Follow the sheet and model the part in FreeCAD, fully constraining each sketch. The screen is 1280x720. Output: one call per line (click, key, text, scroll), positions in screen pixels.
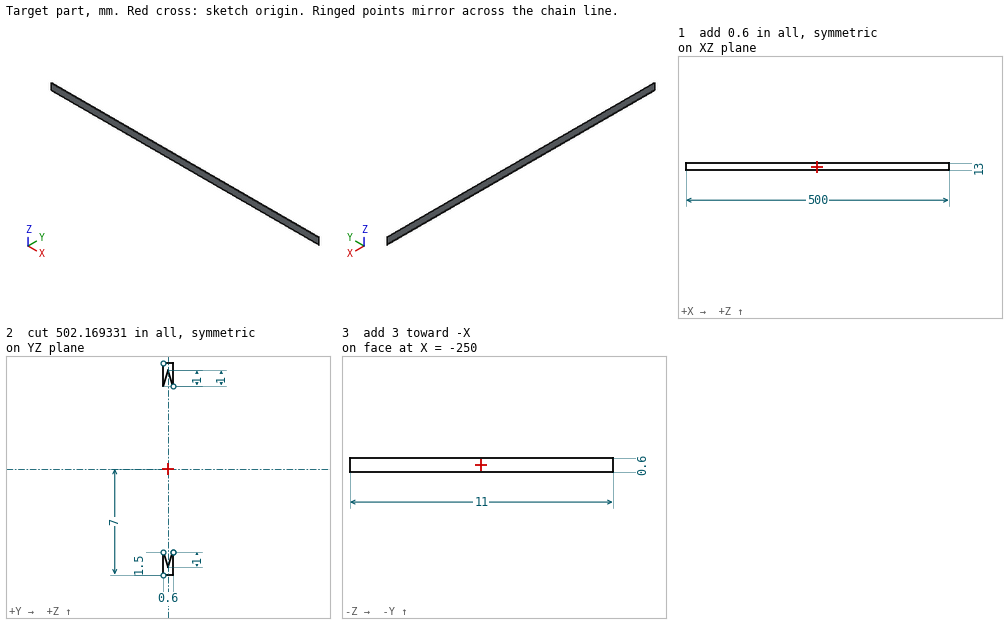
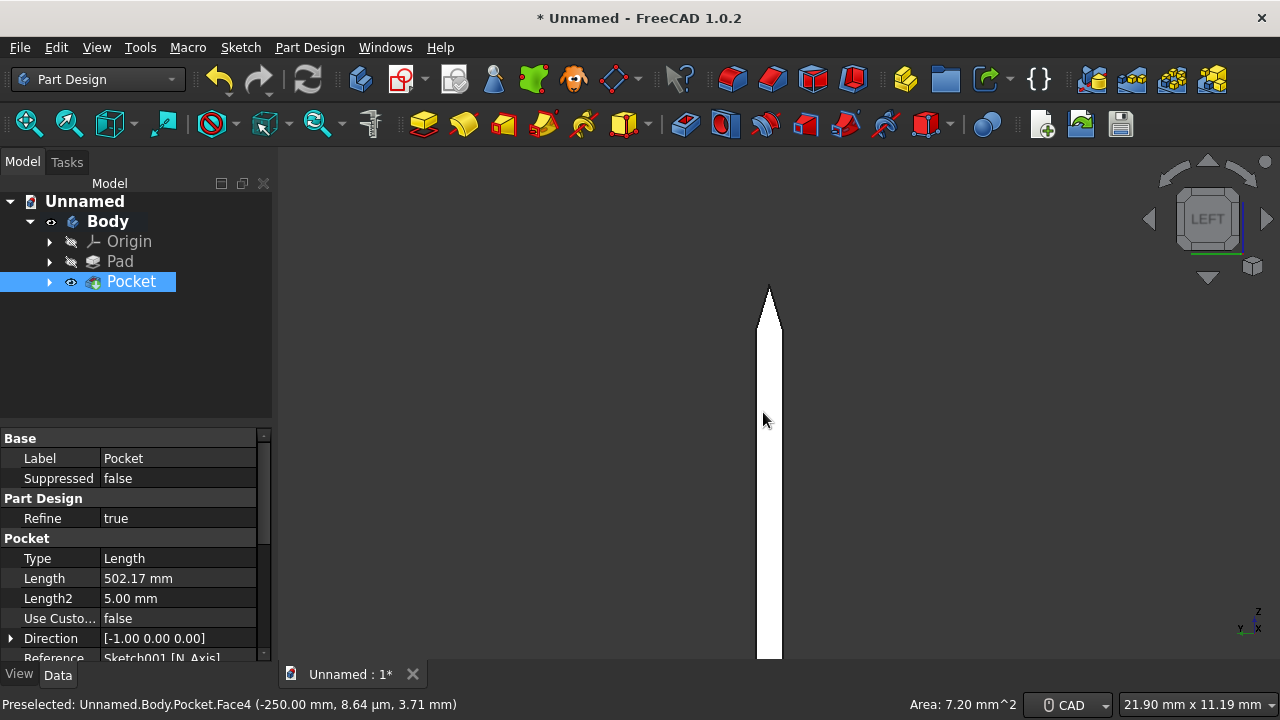
click(402, 80)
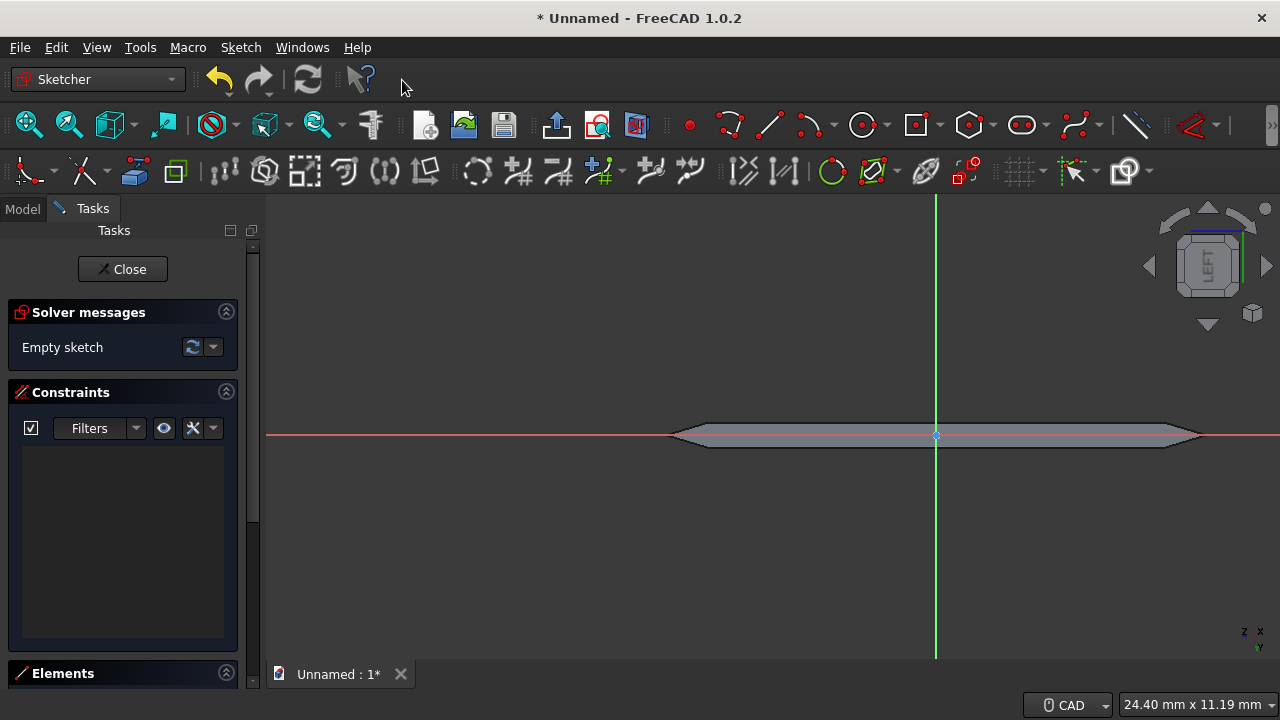
scroll(294, 387, down, 1)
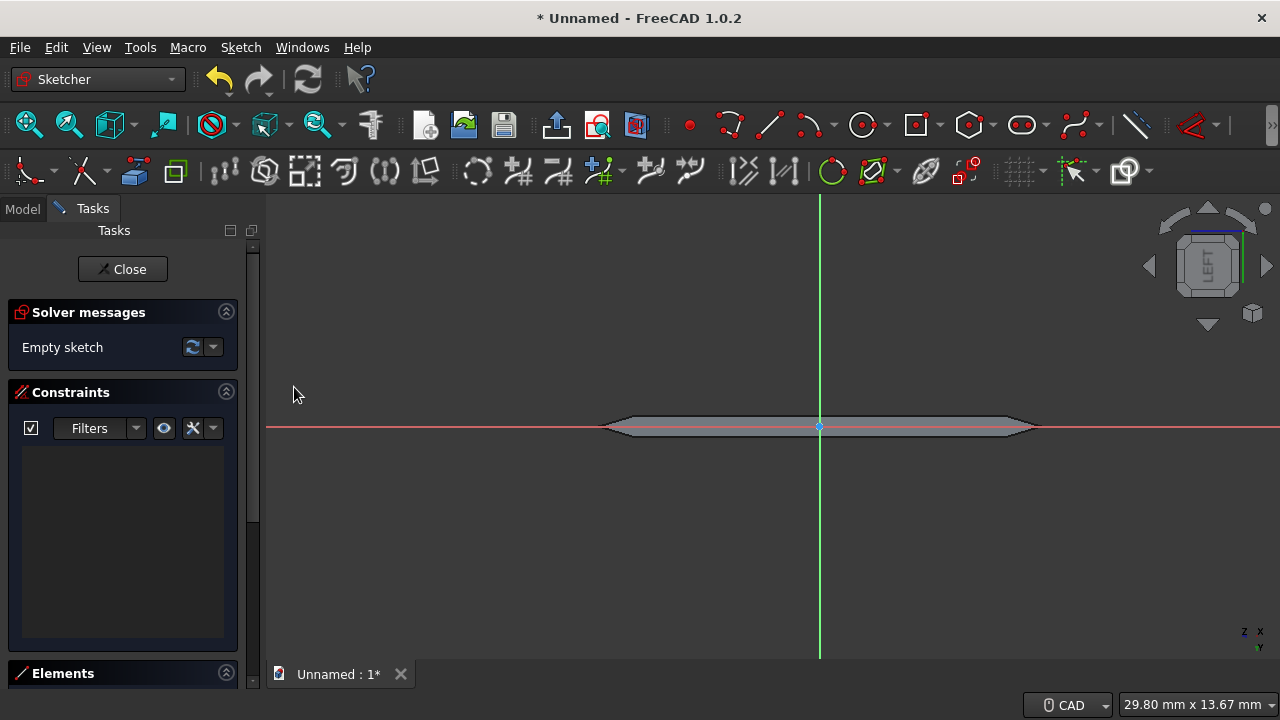
scroll(1055, 427, up, 2)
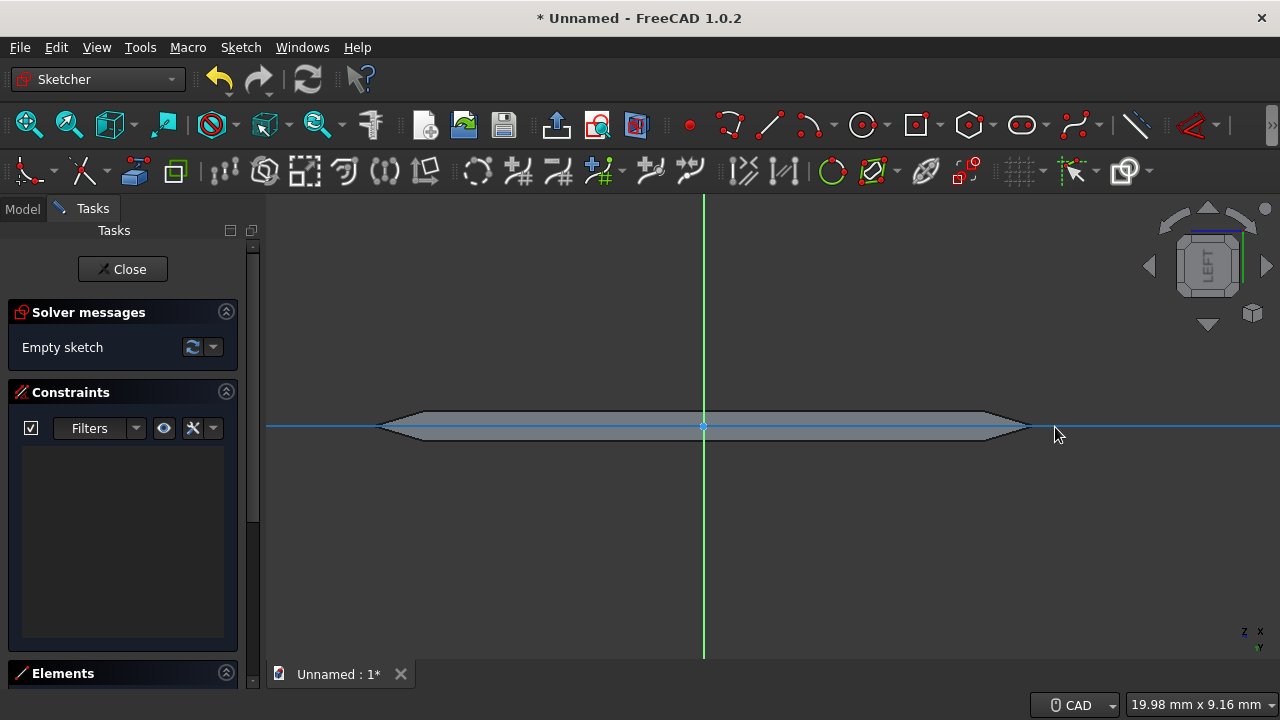
click(916, 126)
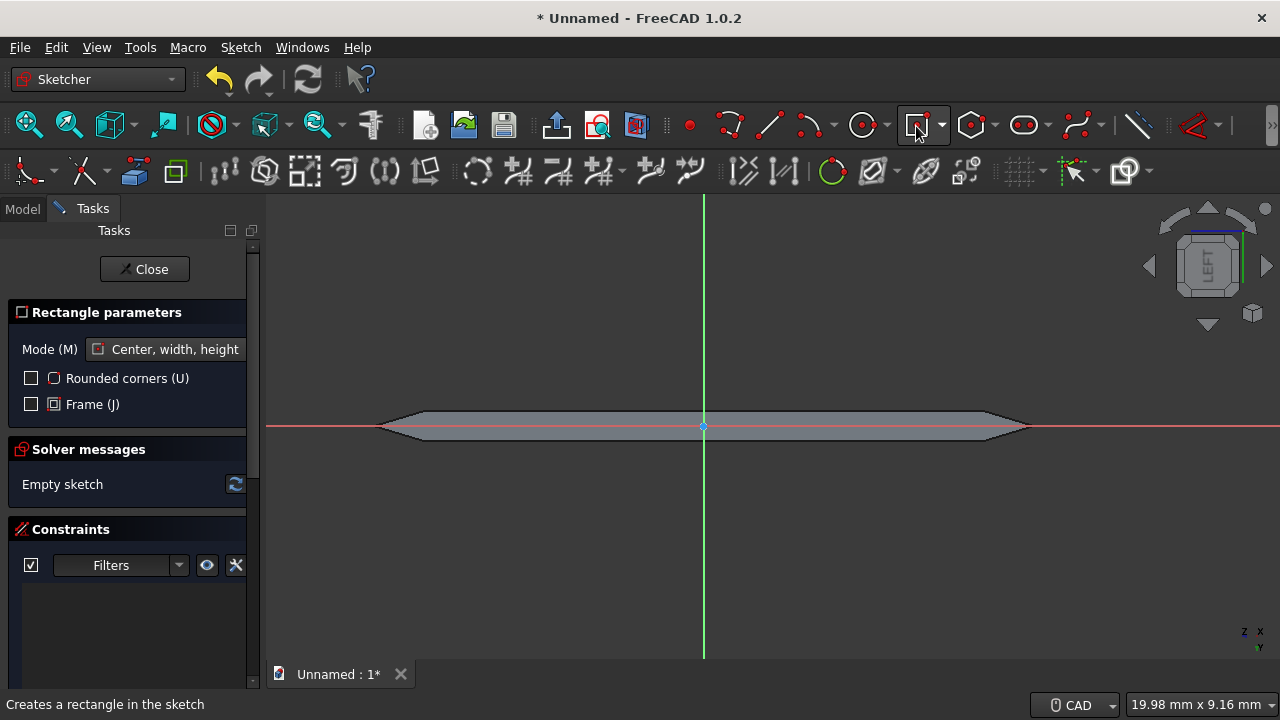
click(704, 426)
move(983, 411)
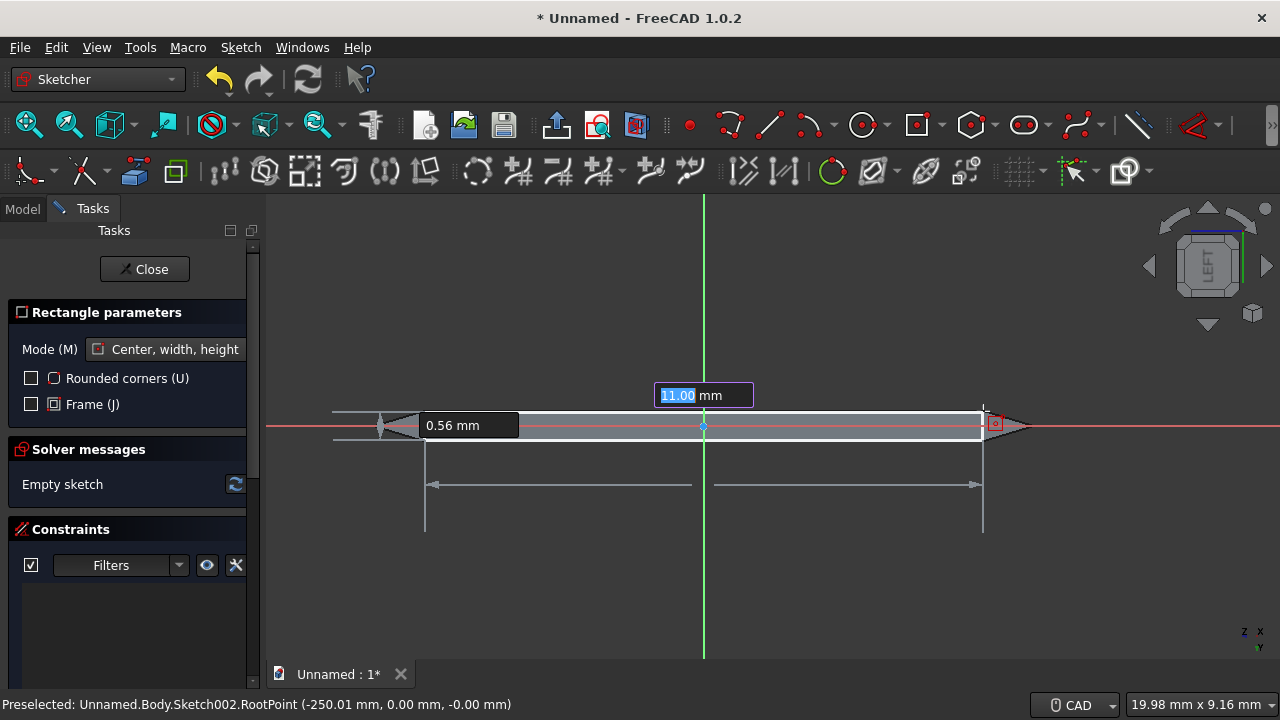
text(11)
key(Tab)
text(0.6)
key(Return)
key(Escape)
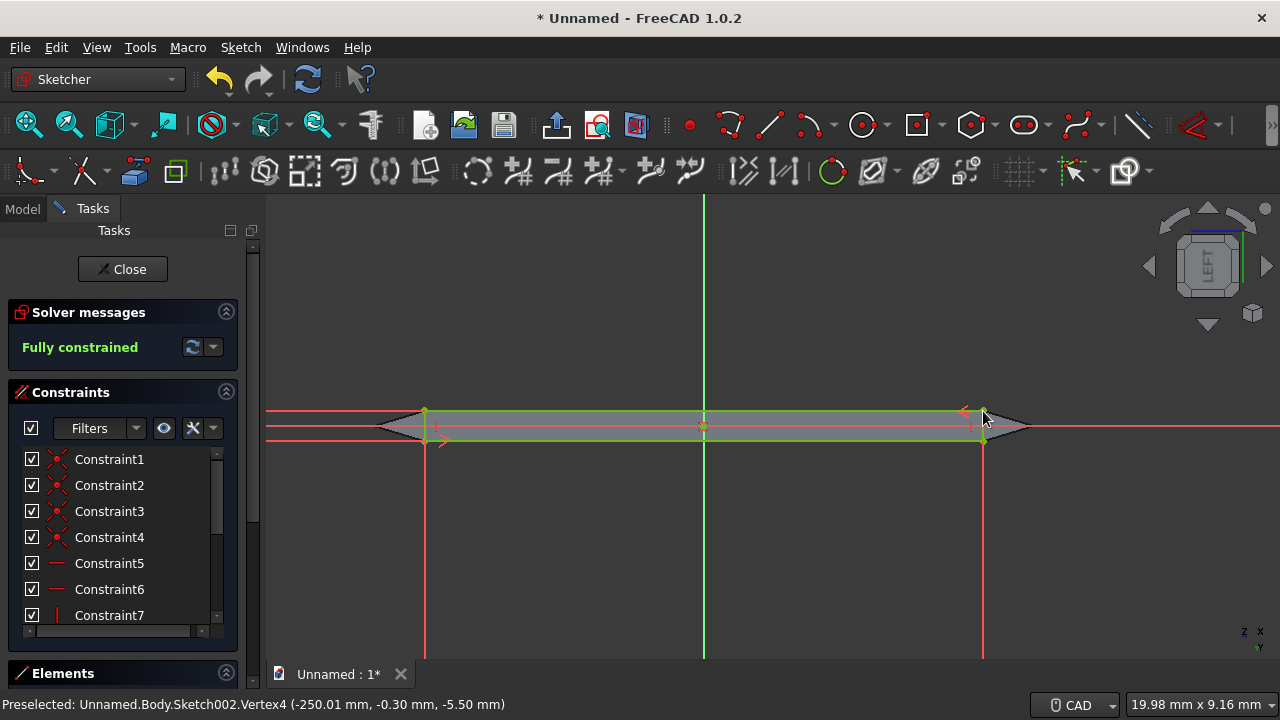
click(123, 269)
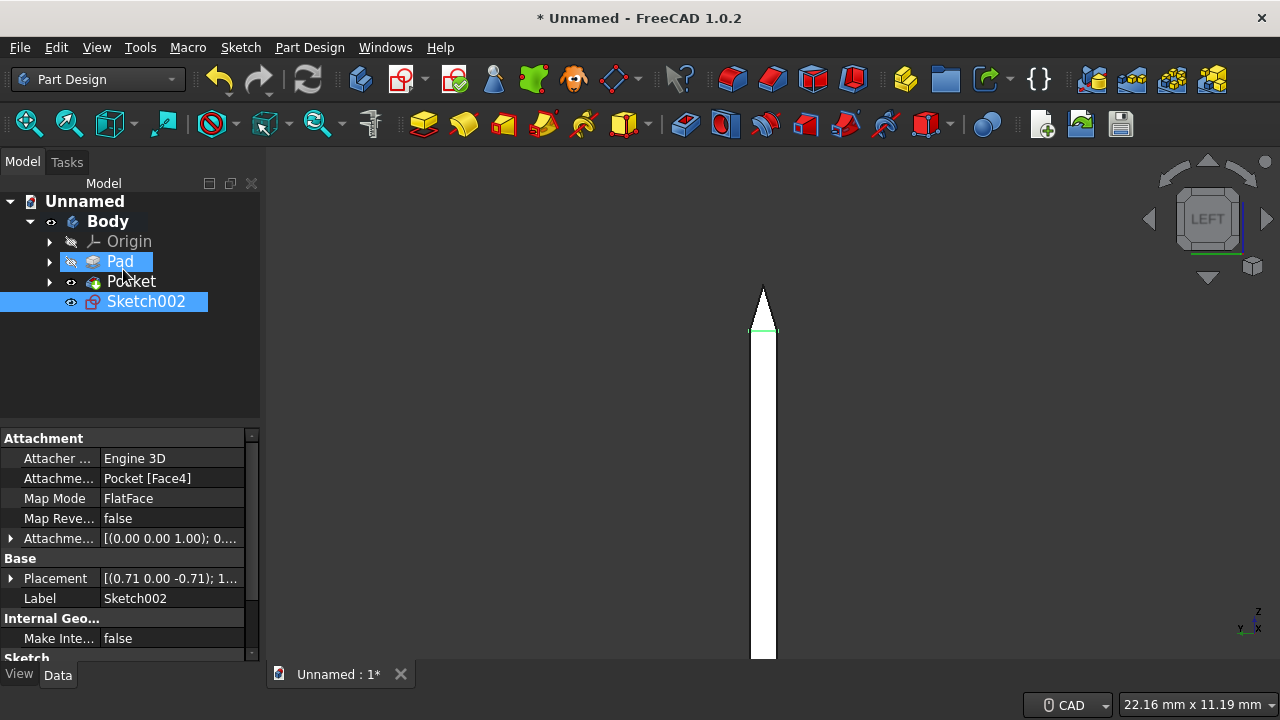
click(424, 124)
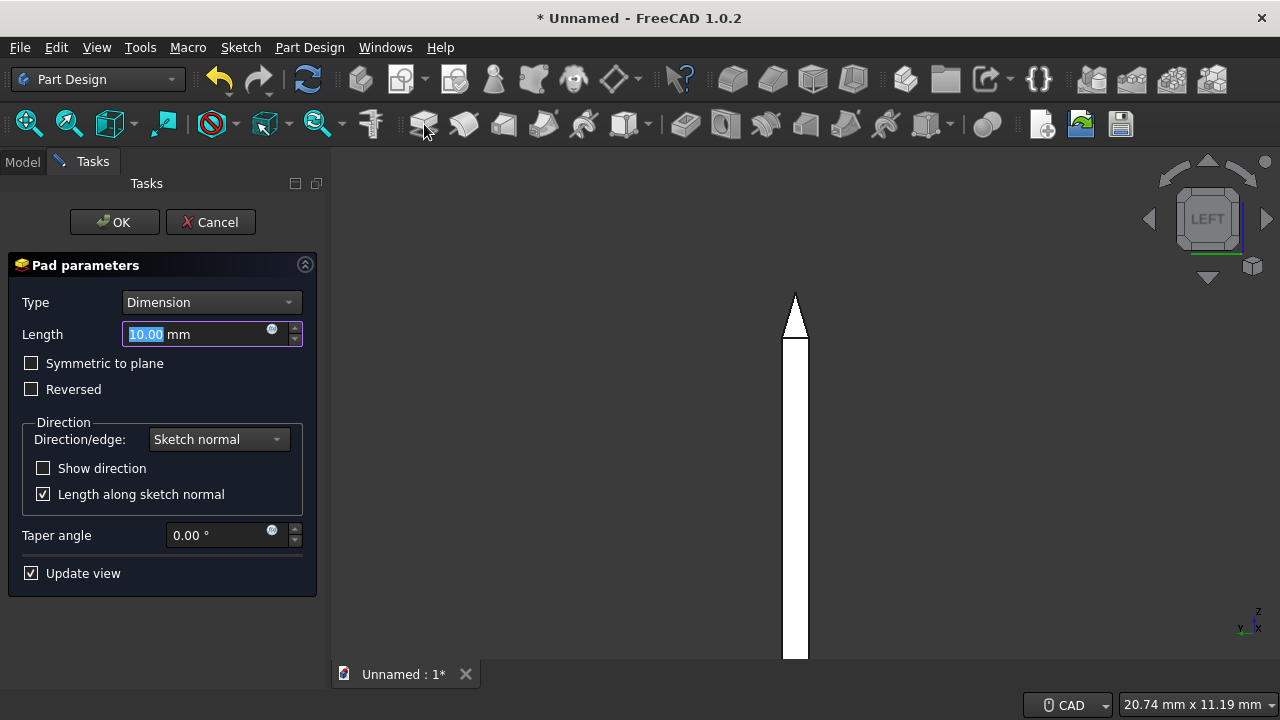
text(3)
key(Tab)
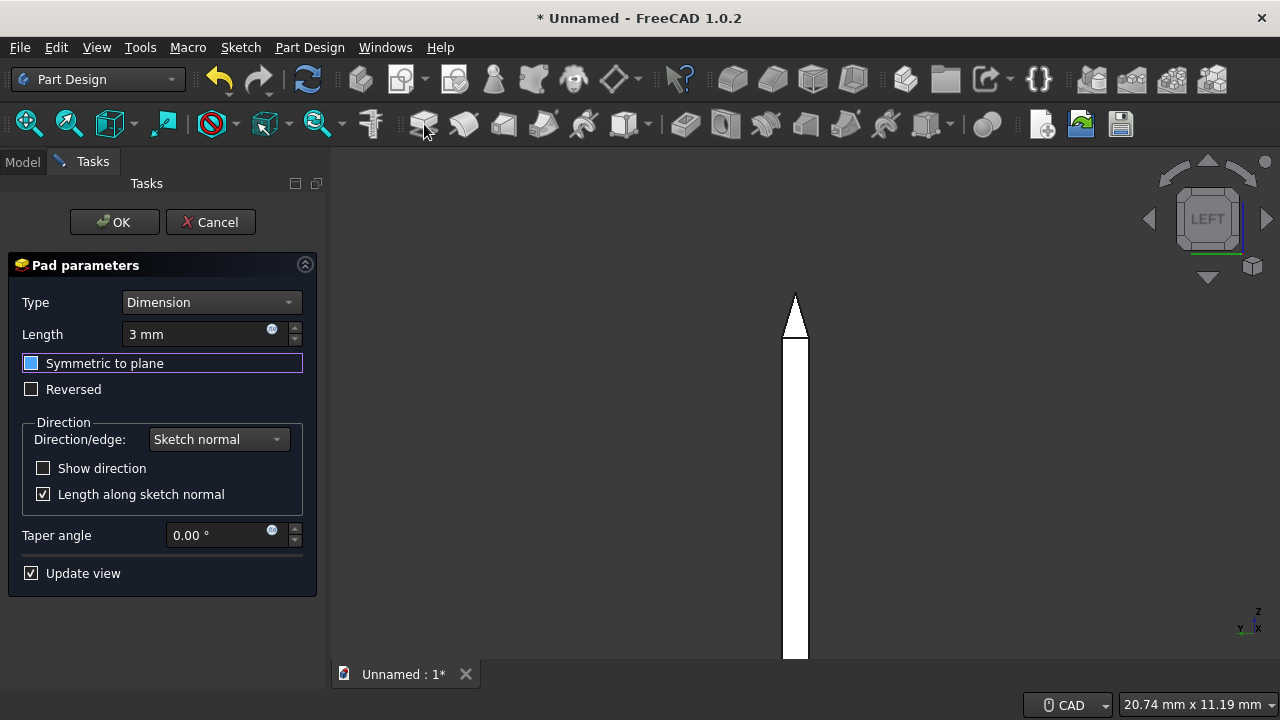
click(115, 222)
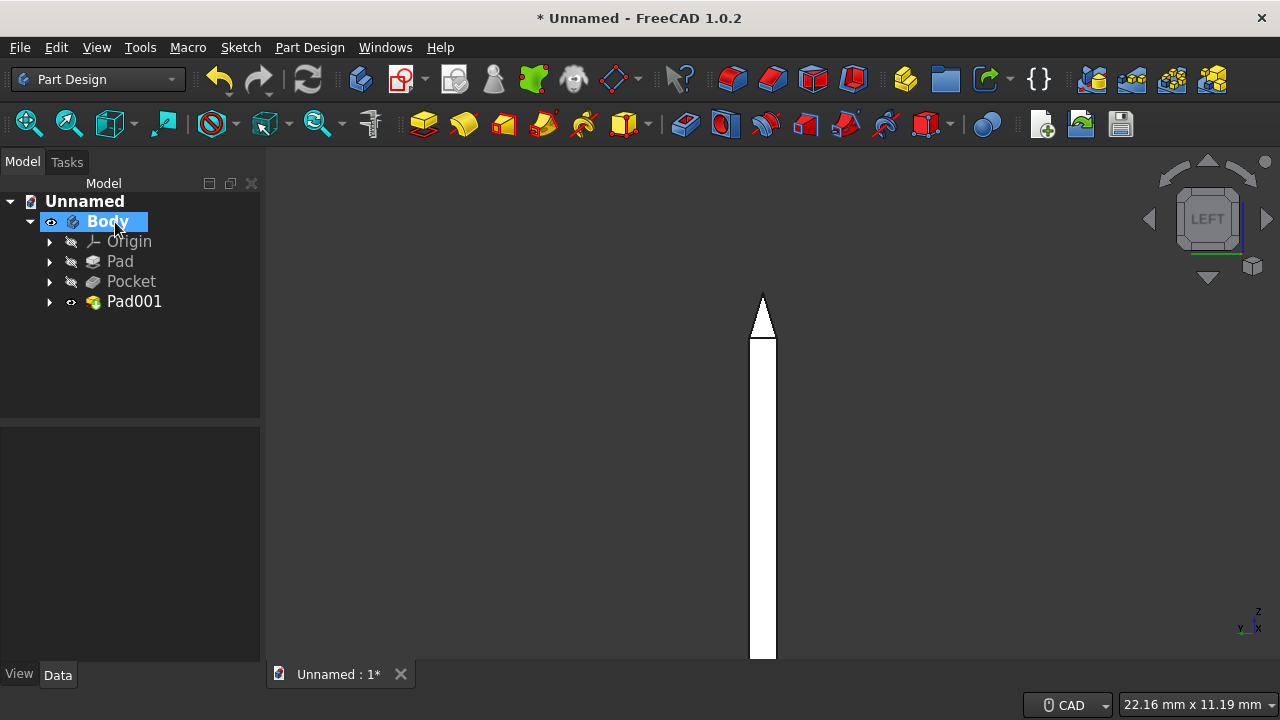
key(0)